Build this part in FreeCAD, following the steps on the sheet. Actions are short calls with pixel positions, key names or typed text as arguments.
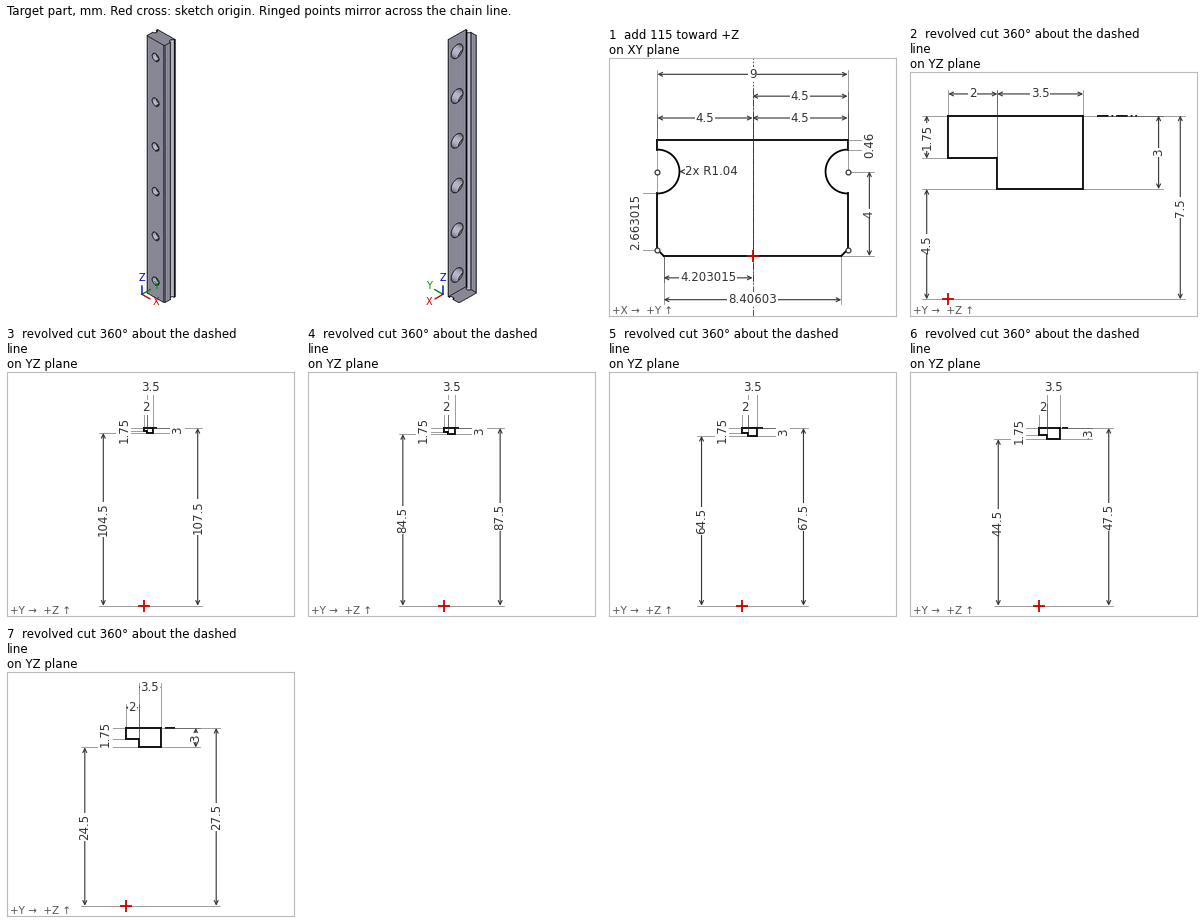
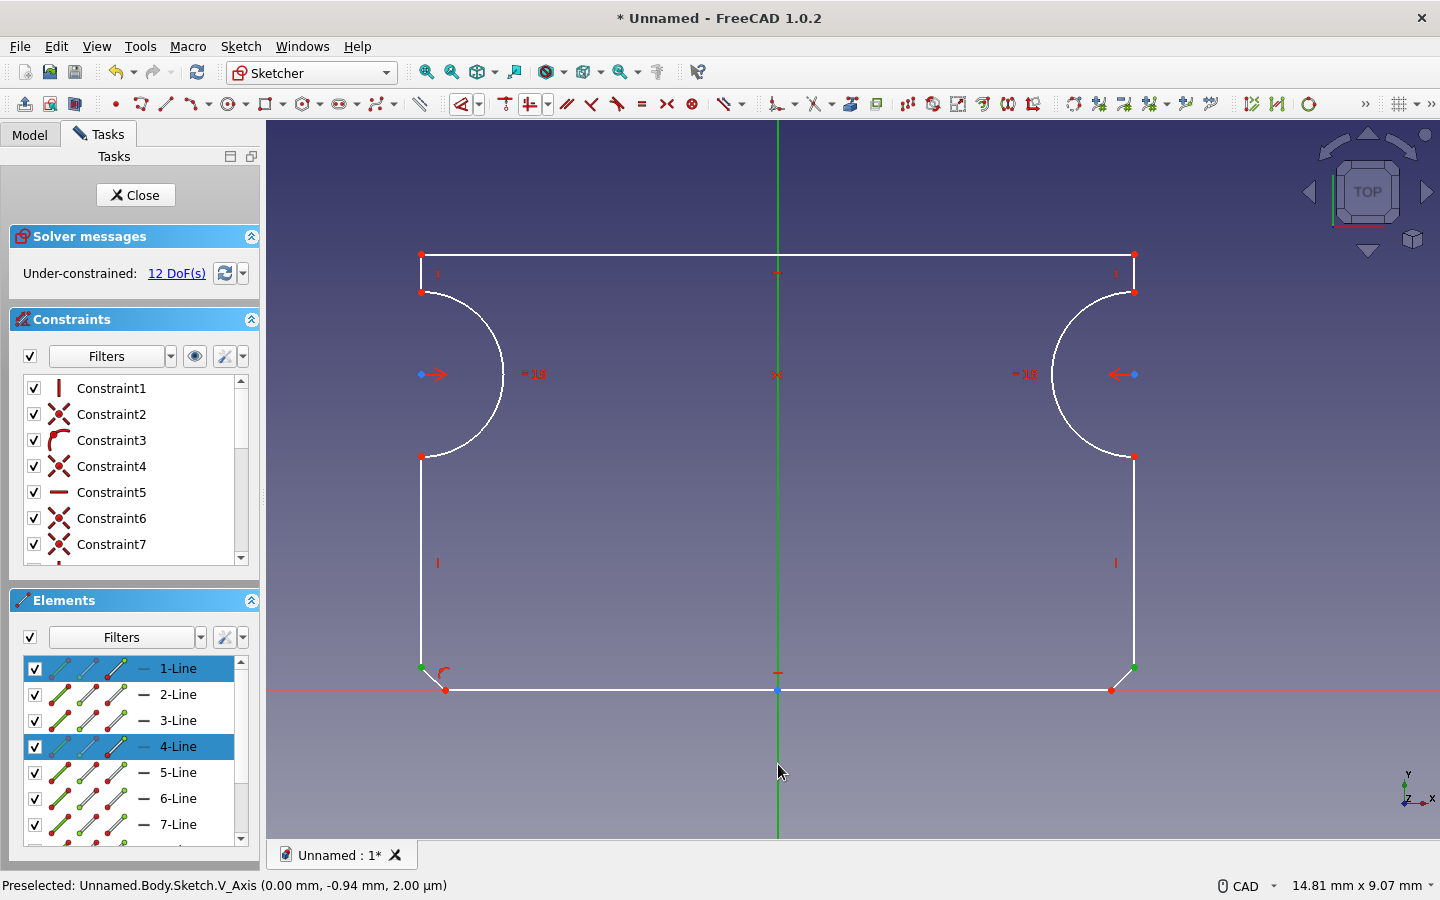
key(s)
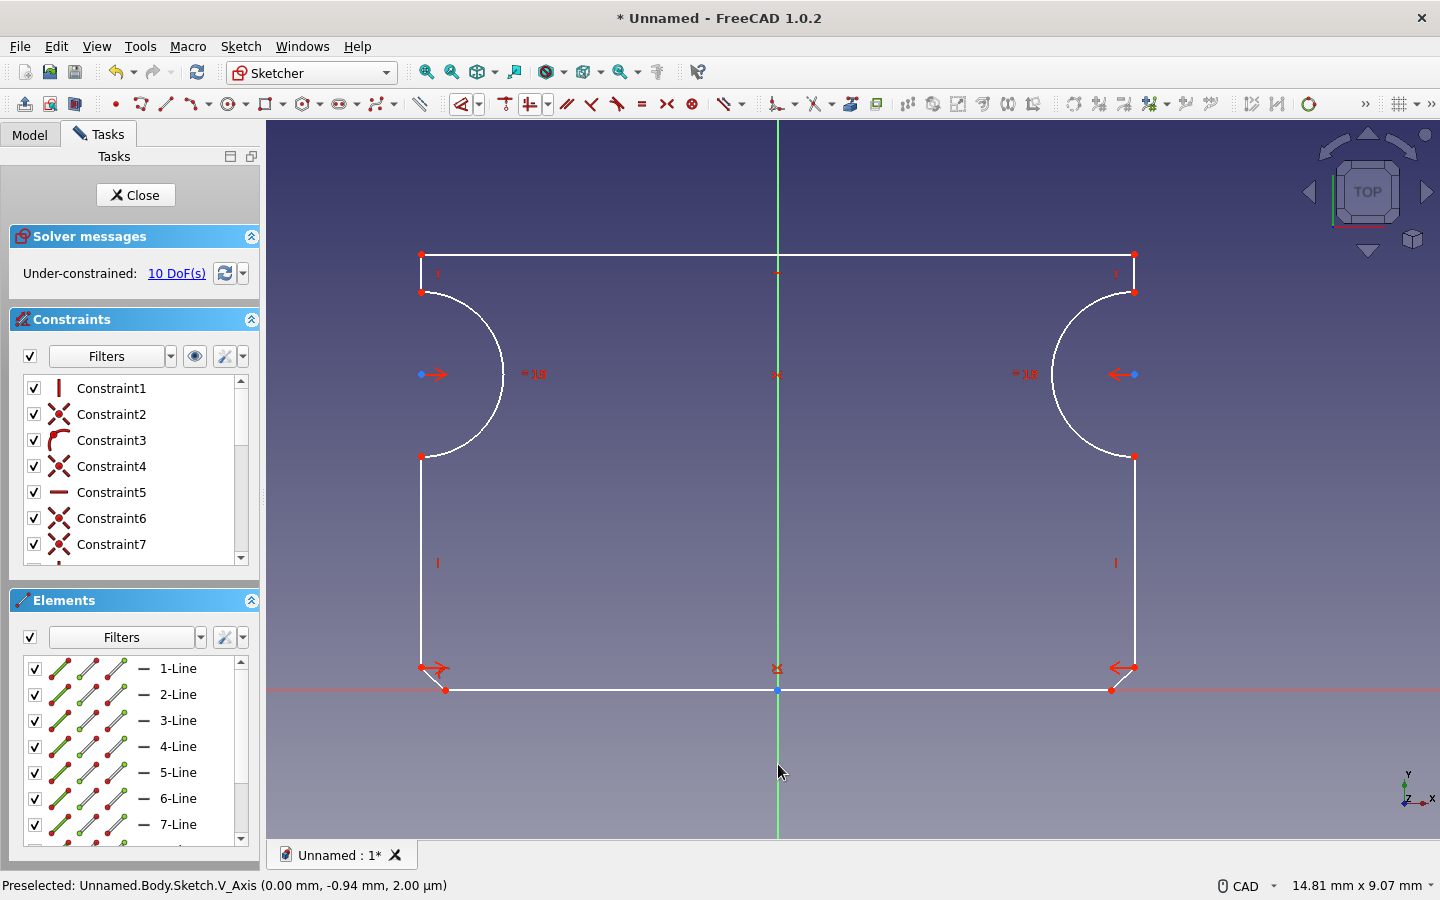
key(d)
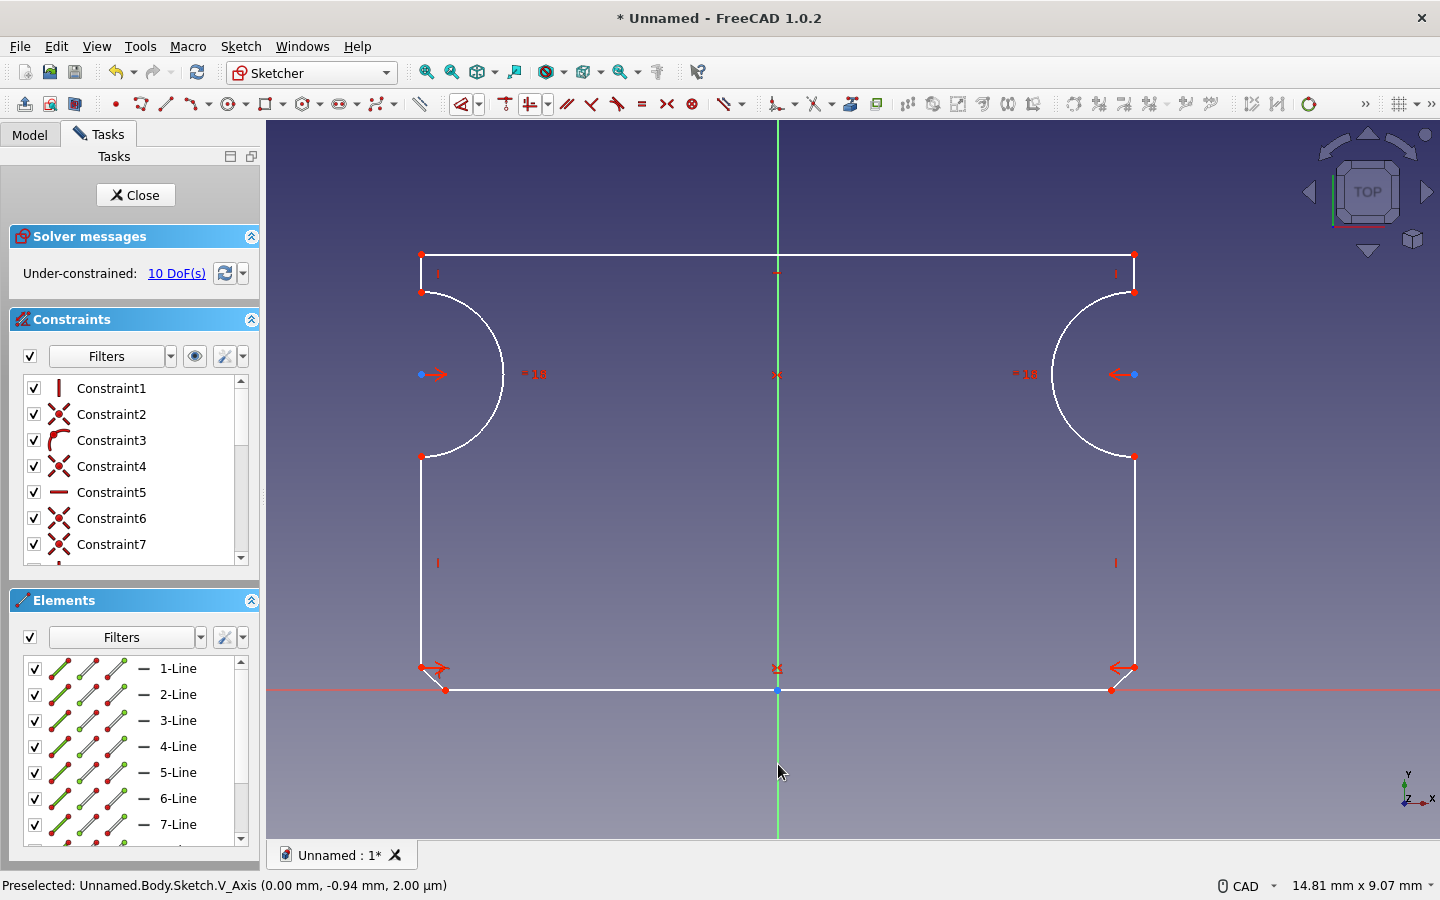
click(1068, 326)
click(1042, 307)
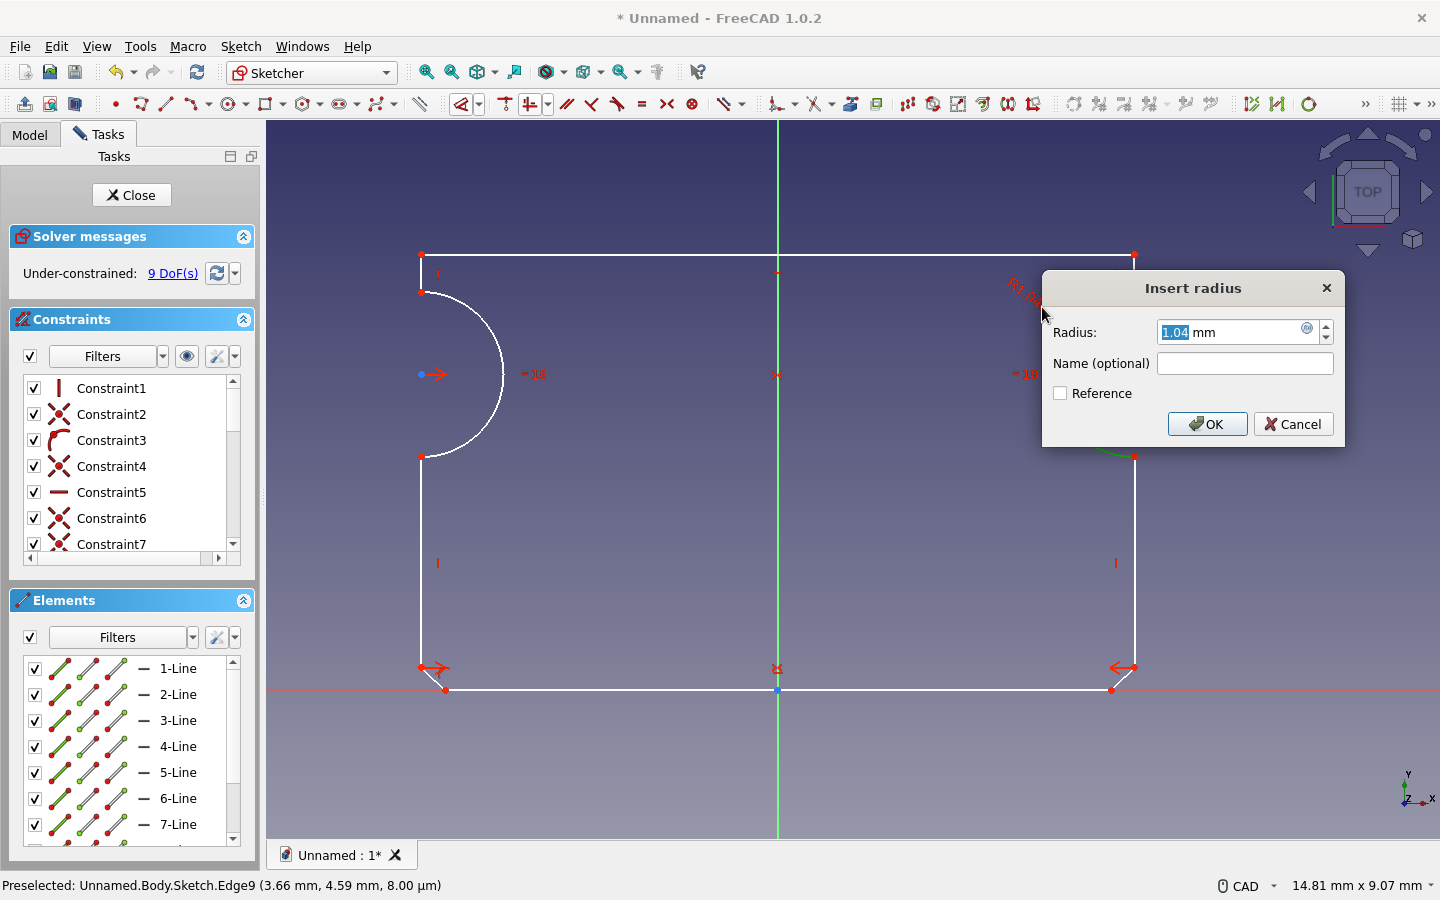
text(1.04)
key(Return)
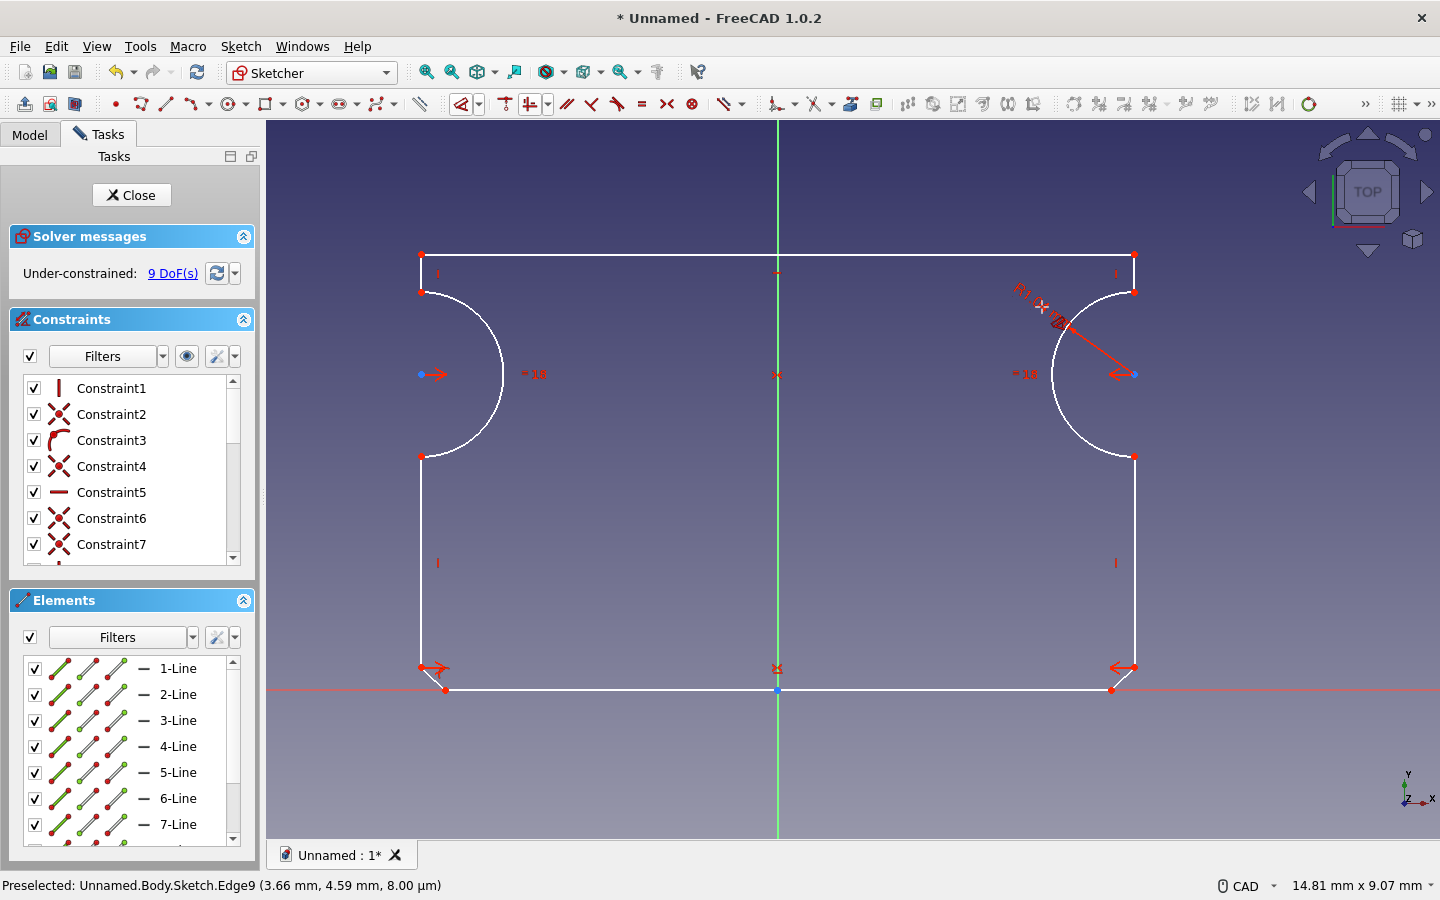
click(920, 255)
click(614, 221)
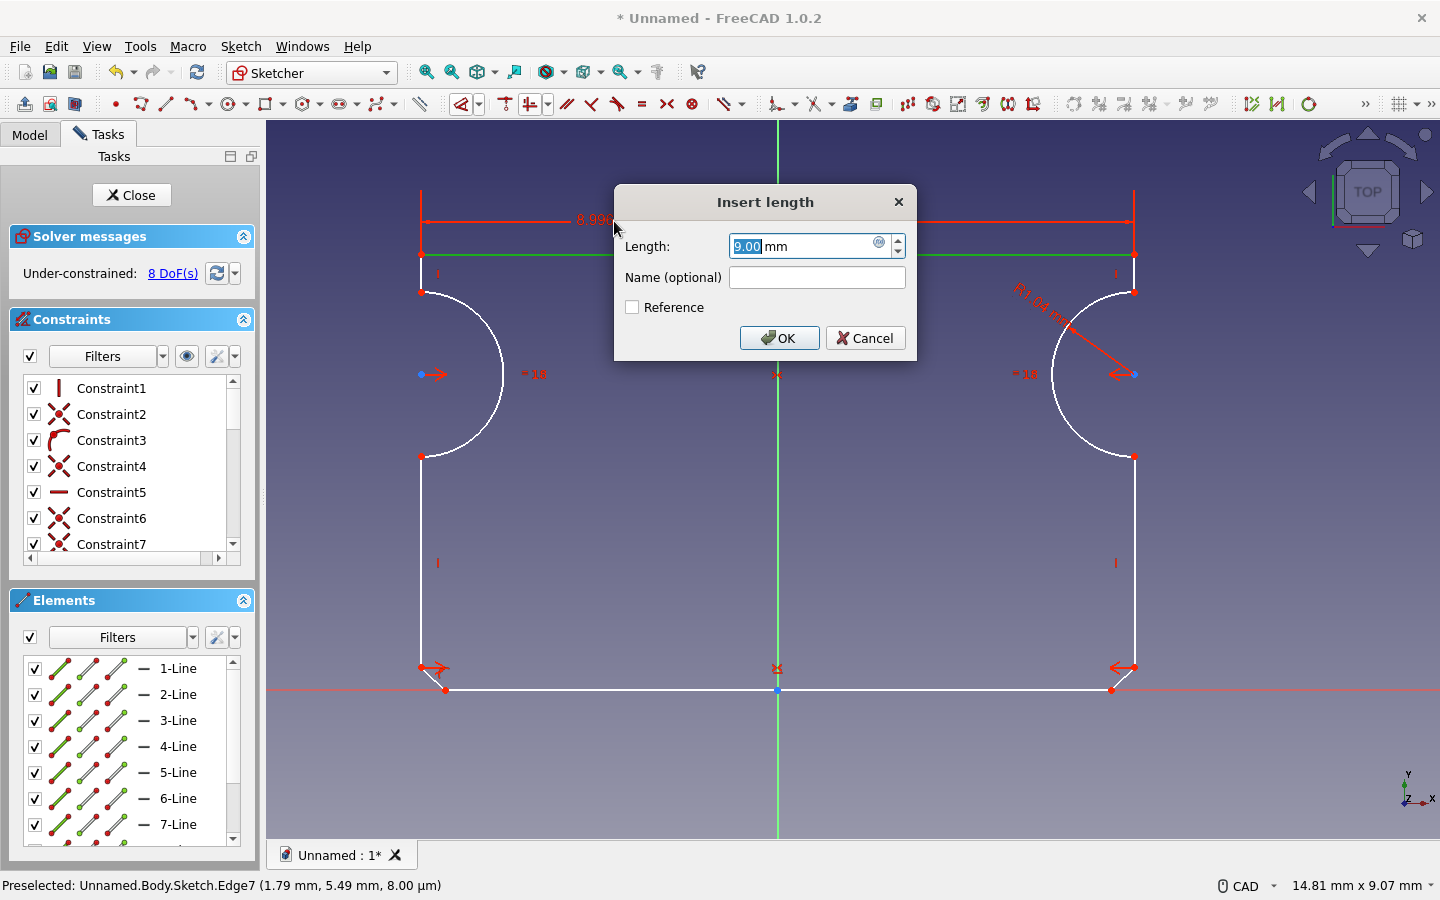
text(9)
key(Return)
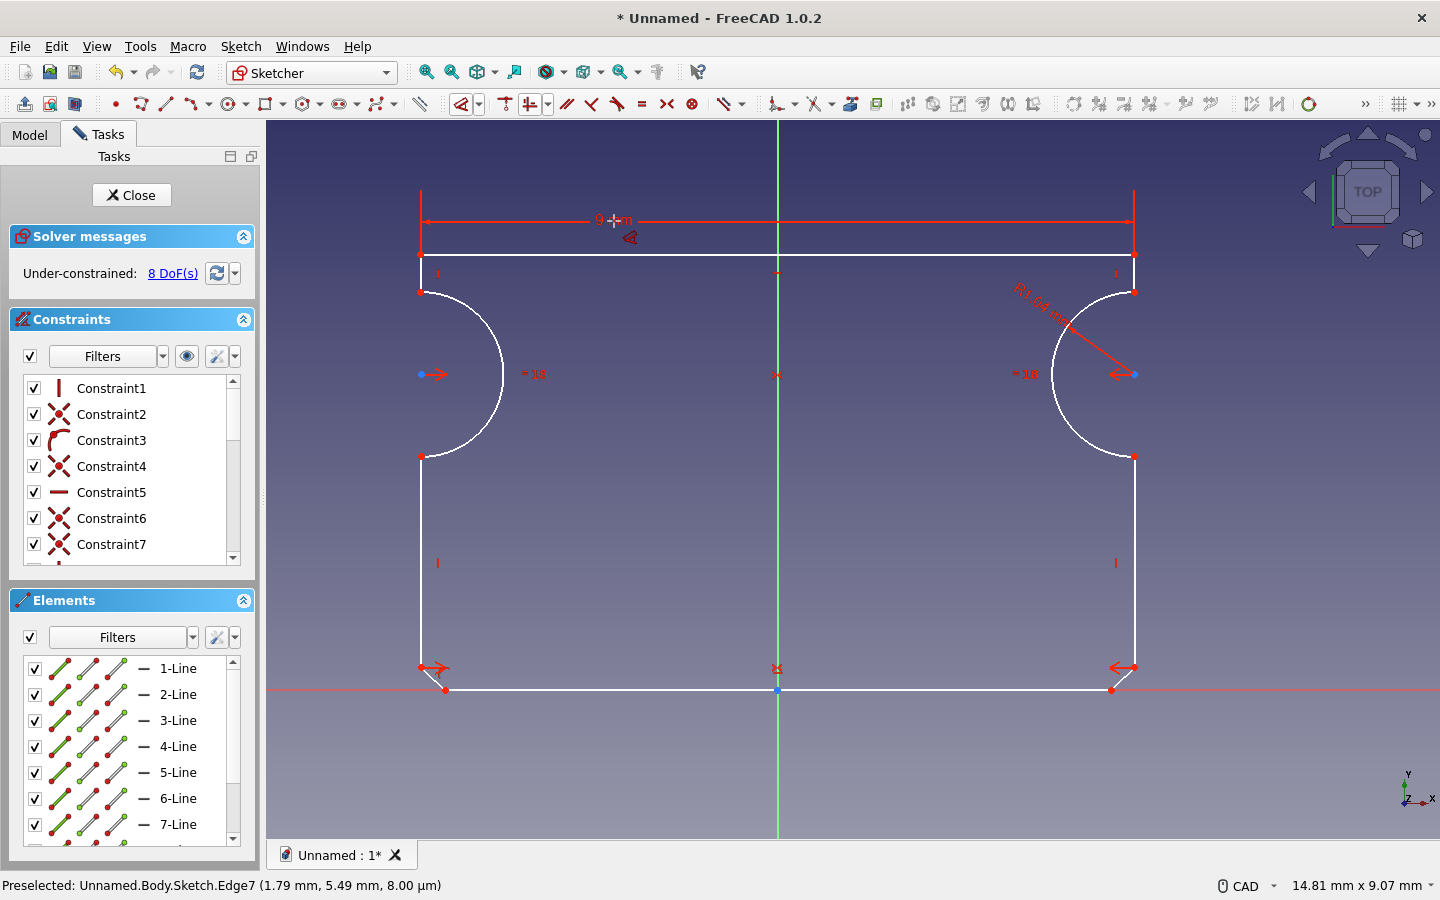
click(1135, 374)
click(1169, 532)